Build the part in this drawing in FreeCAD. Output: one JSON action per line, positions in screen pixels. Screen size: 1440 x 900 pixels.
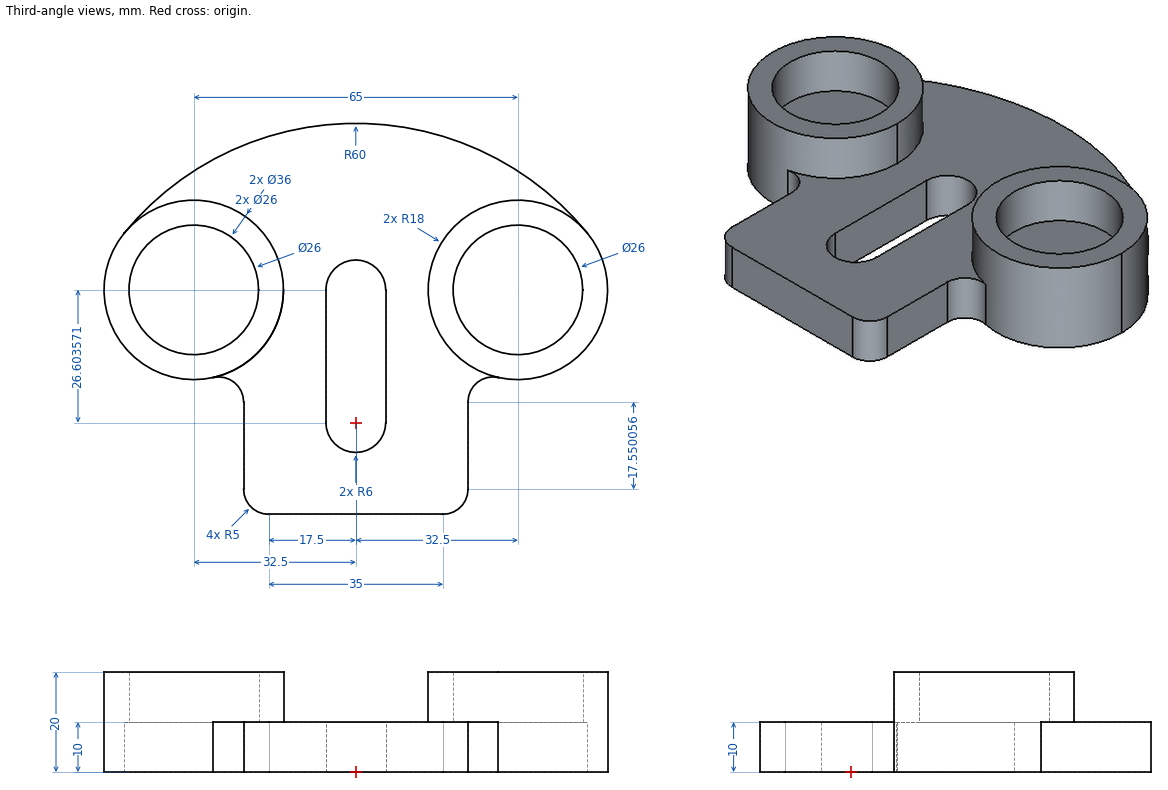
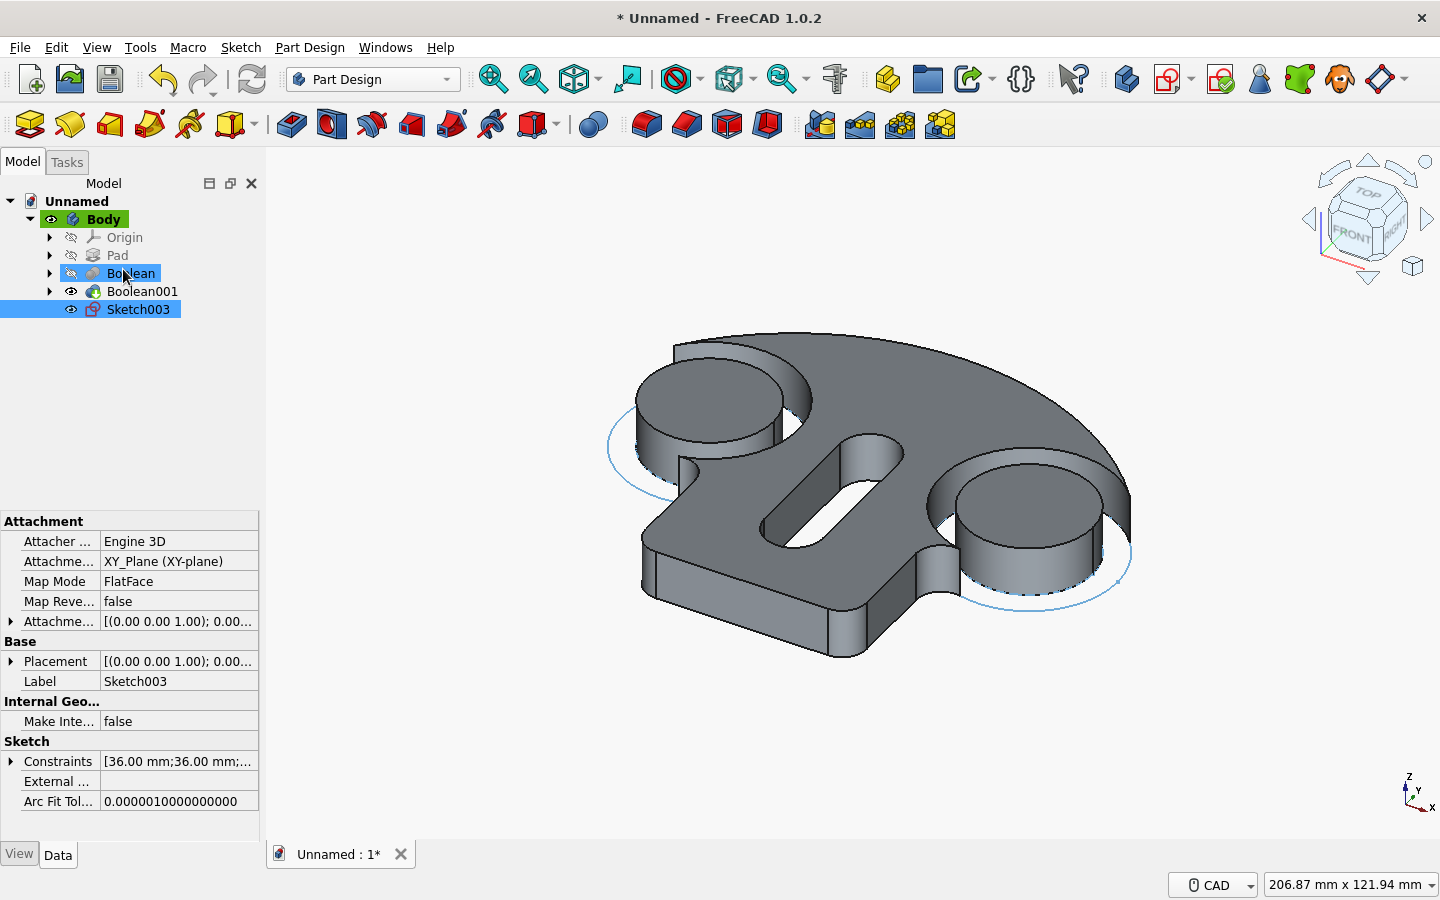
{"action": "left_click", "coordinate": [30, 124]}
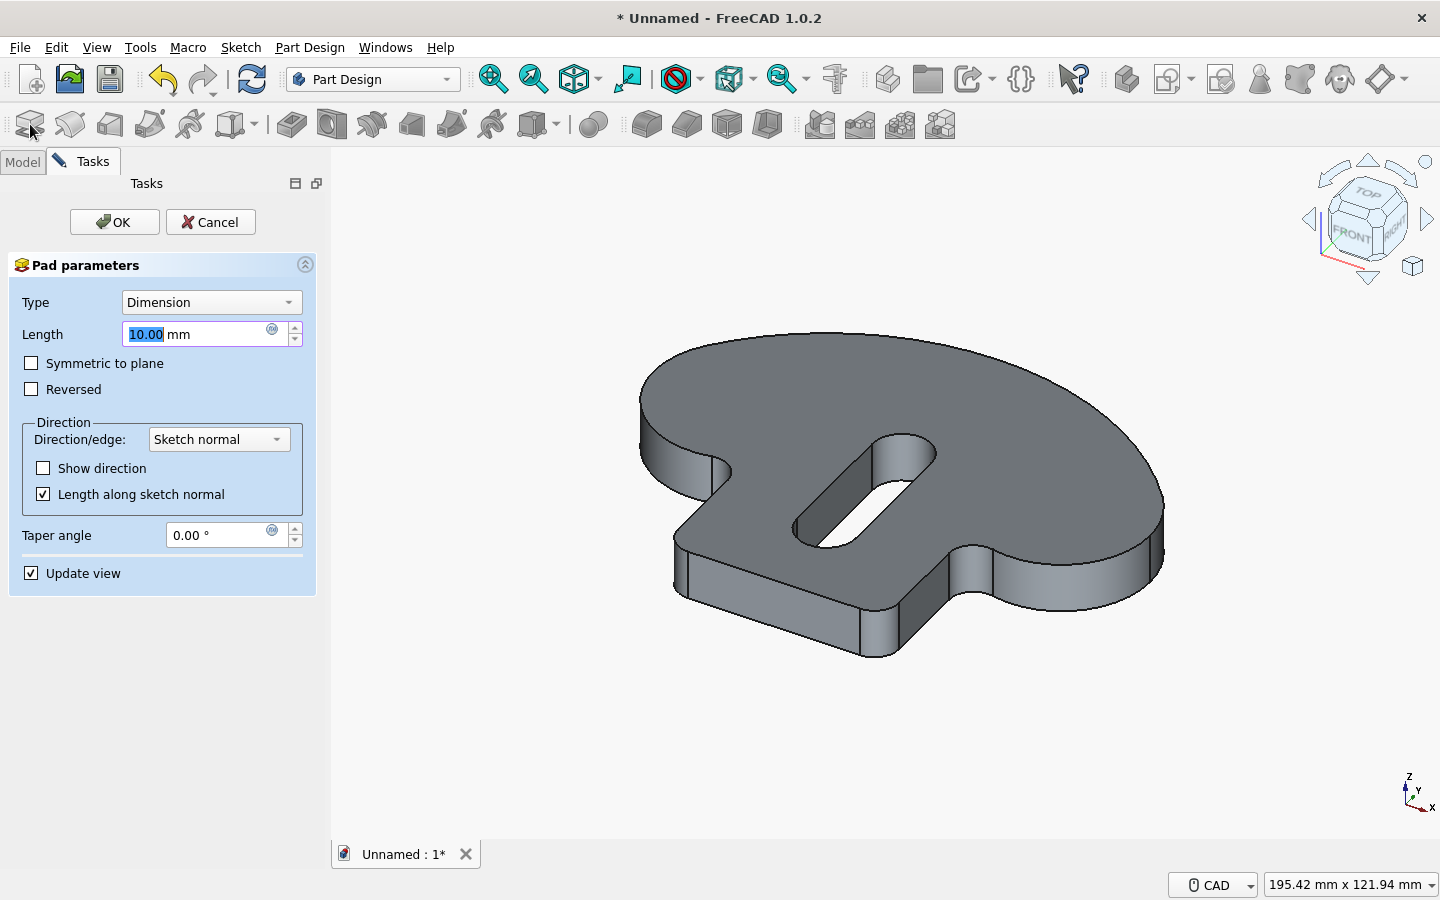
{"action": "type", "text": "20"}
{"action": "key", "text": "Tab"}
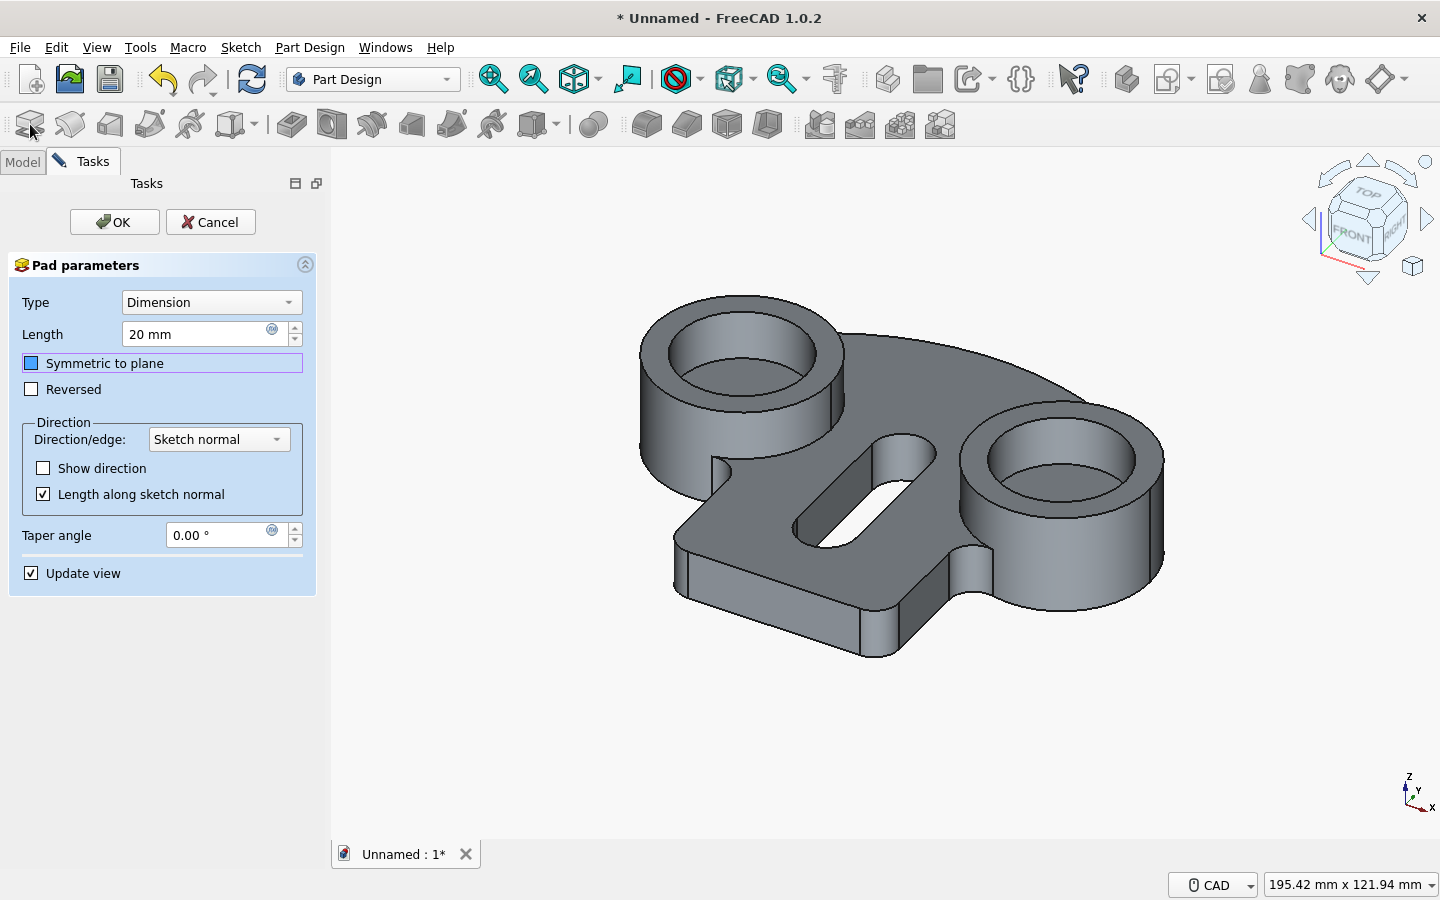
{"action": "left_click", "coordinate": [115, 222]}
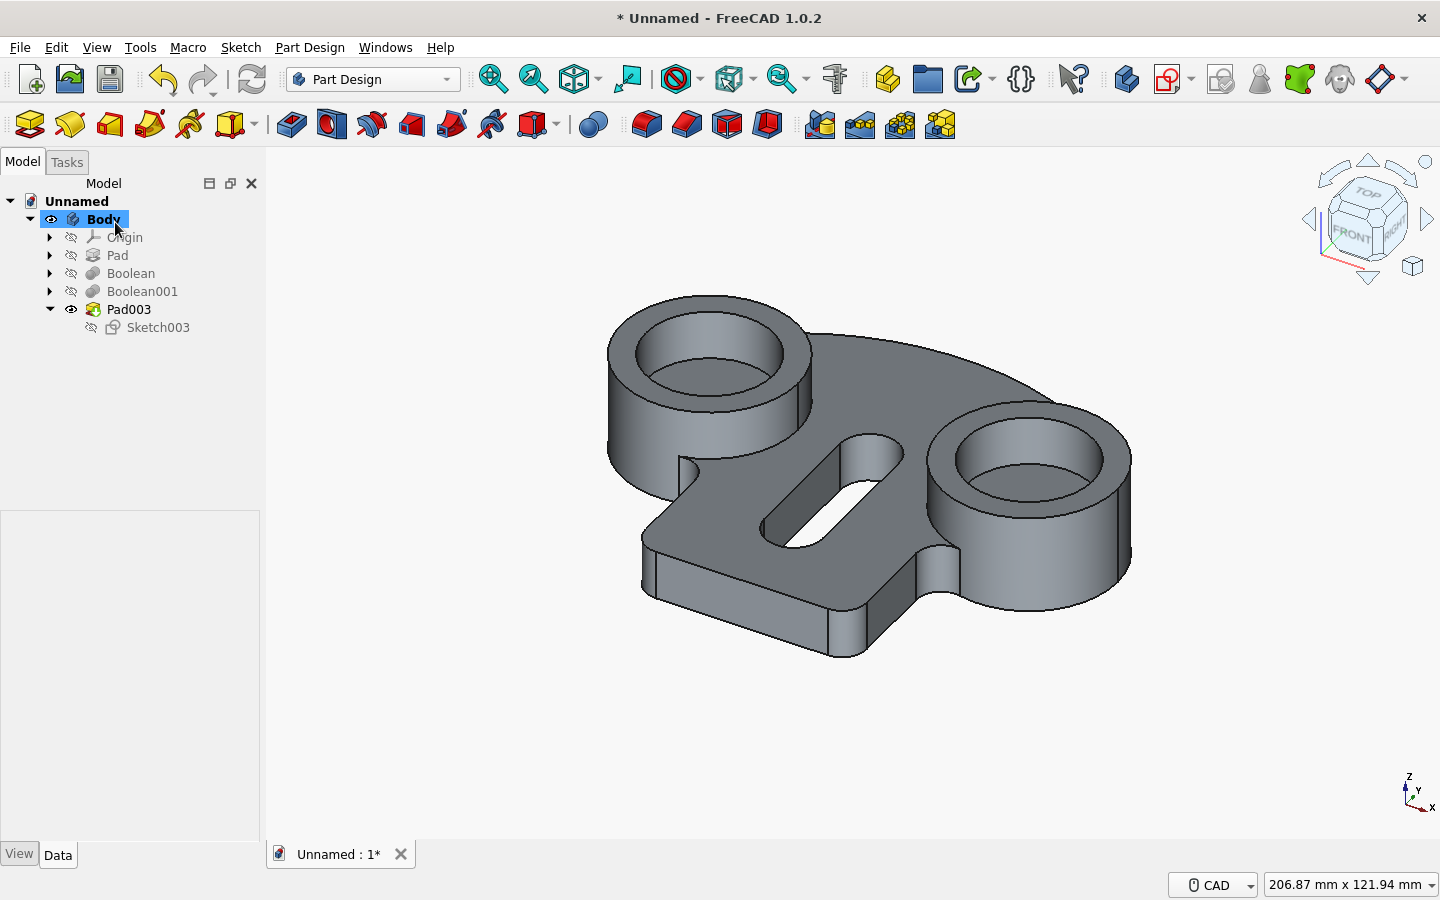
{"action": "key", "text": "0"}